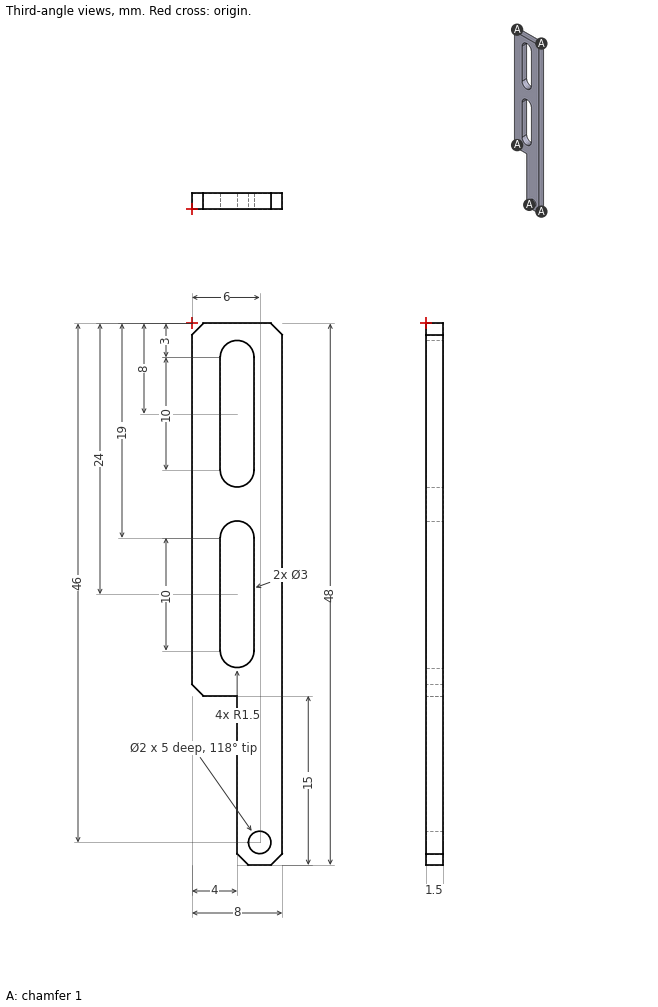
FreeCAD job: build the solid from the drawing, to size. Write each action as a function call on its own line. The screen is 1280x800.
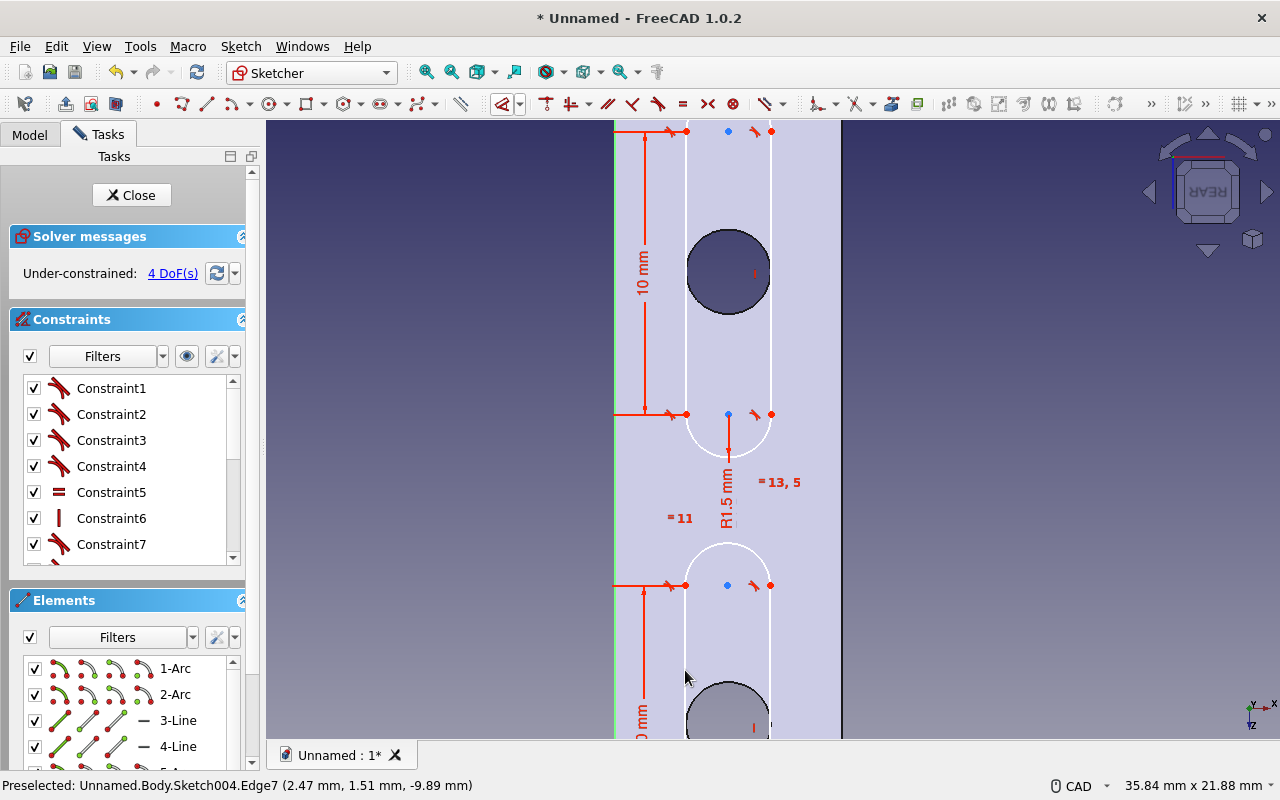
scroll(714, 356, down, 4)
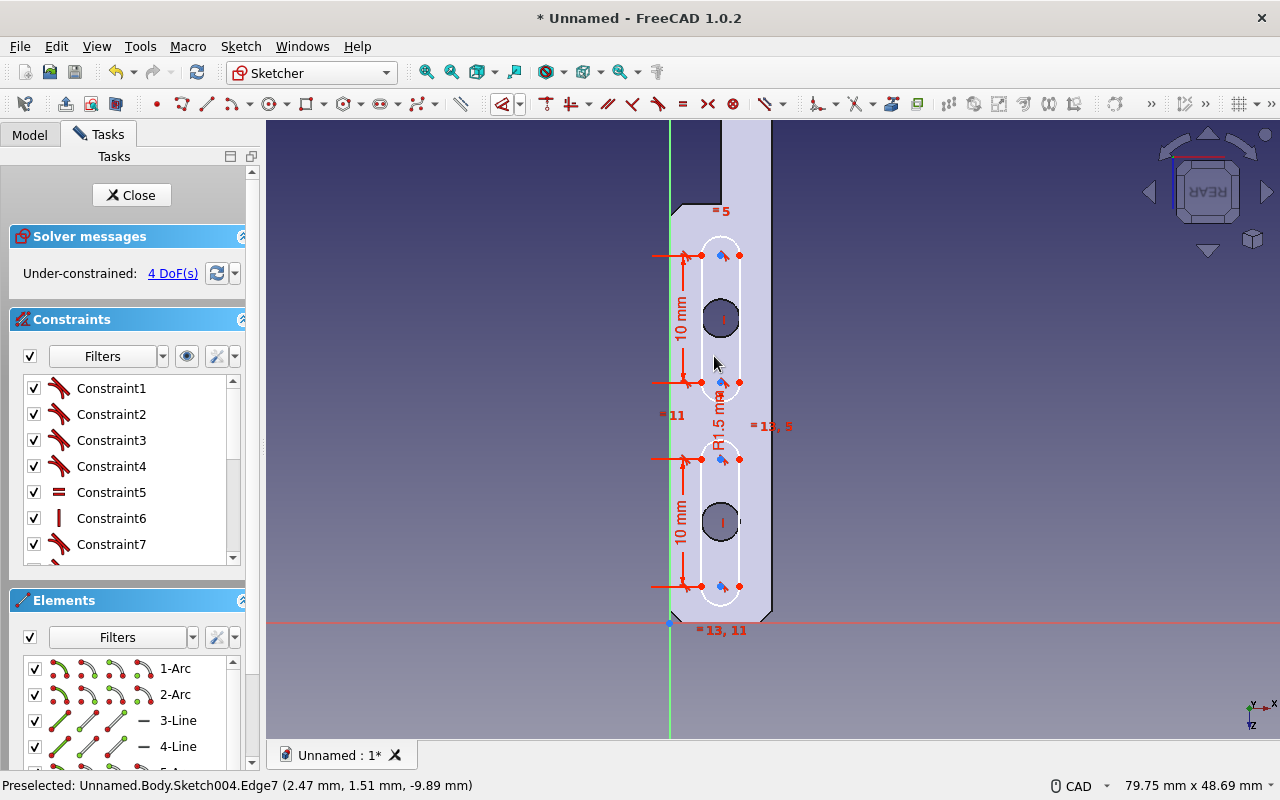
click(701, 587)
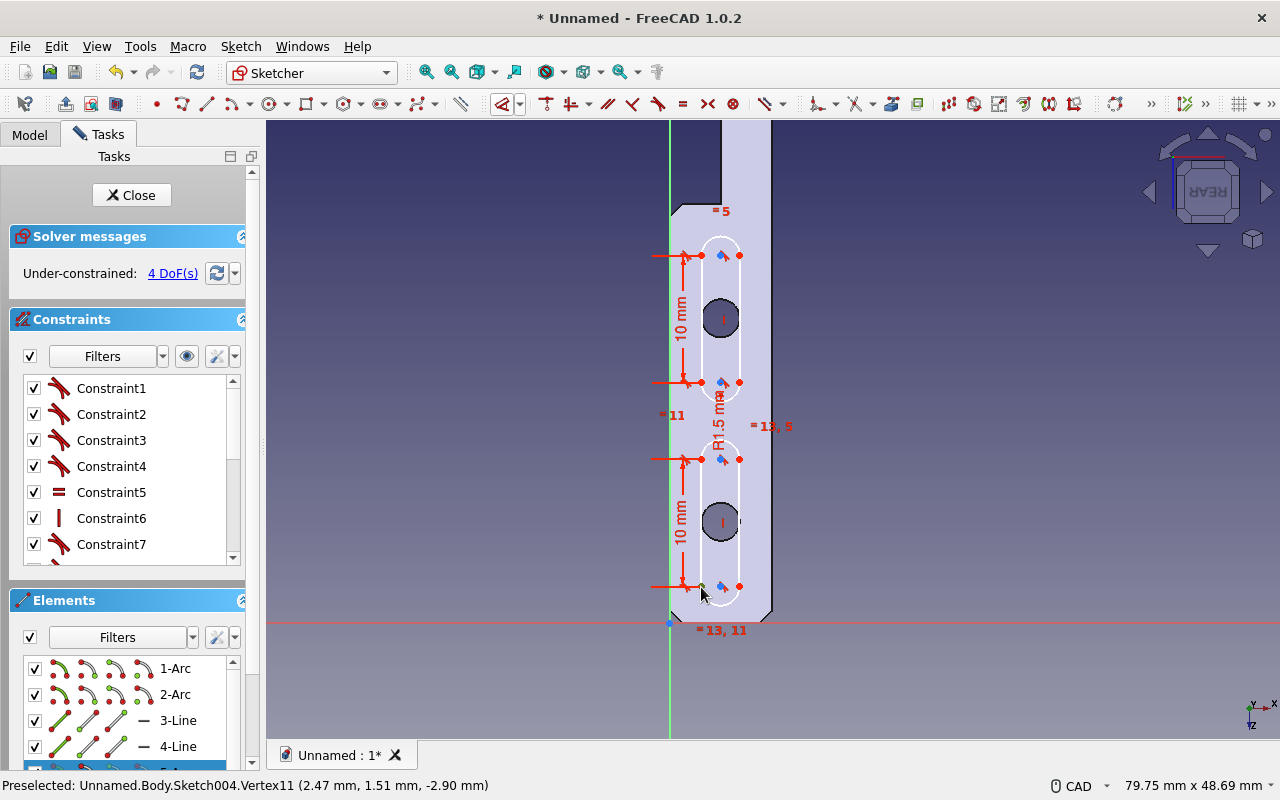
click(520, 104)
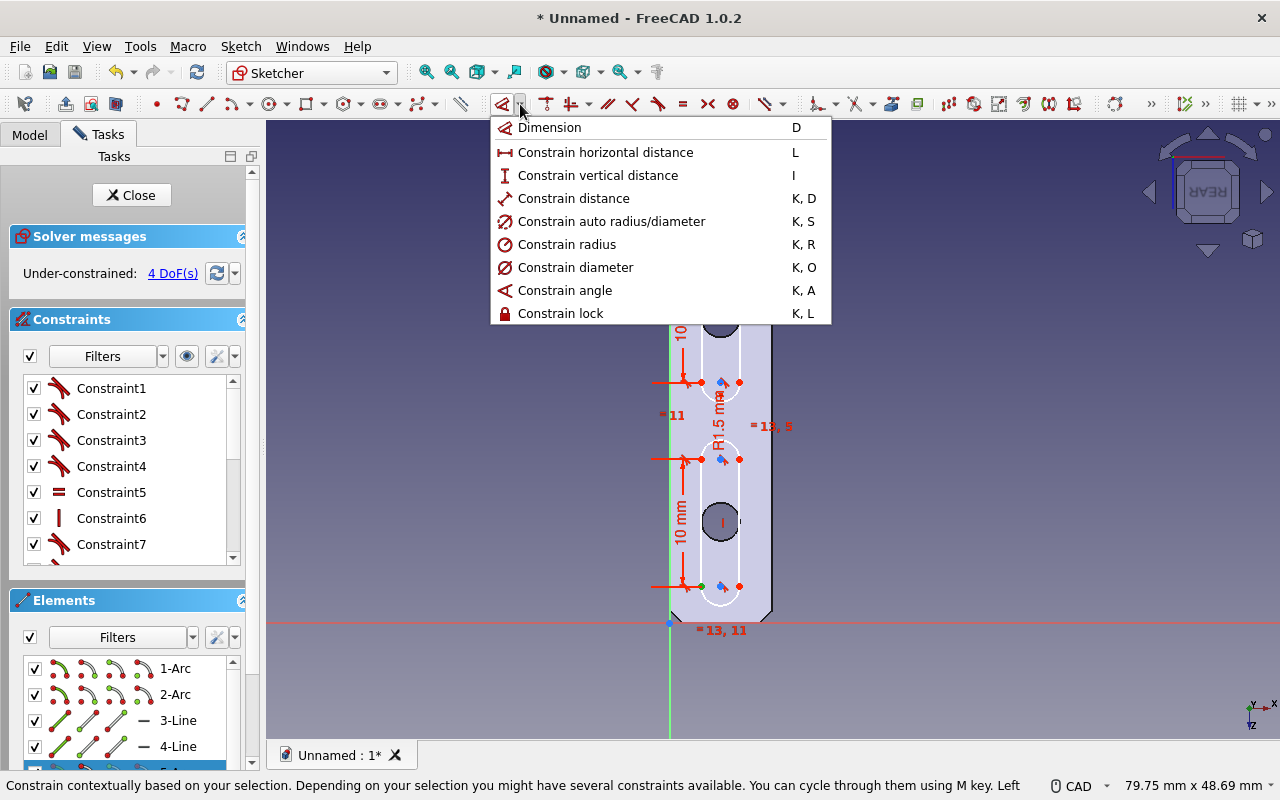
click(661, 176)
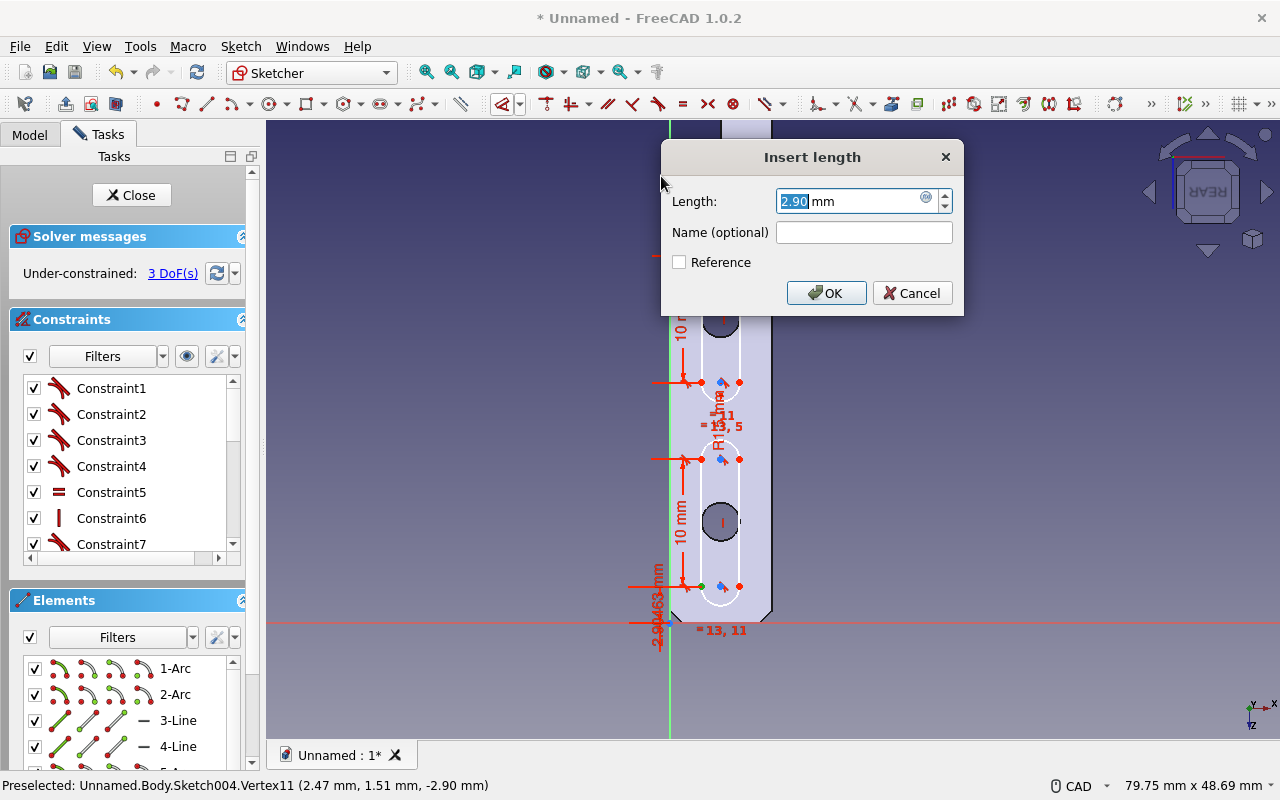
text(3)
key(Return)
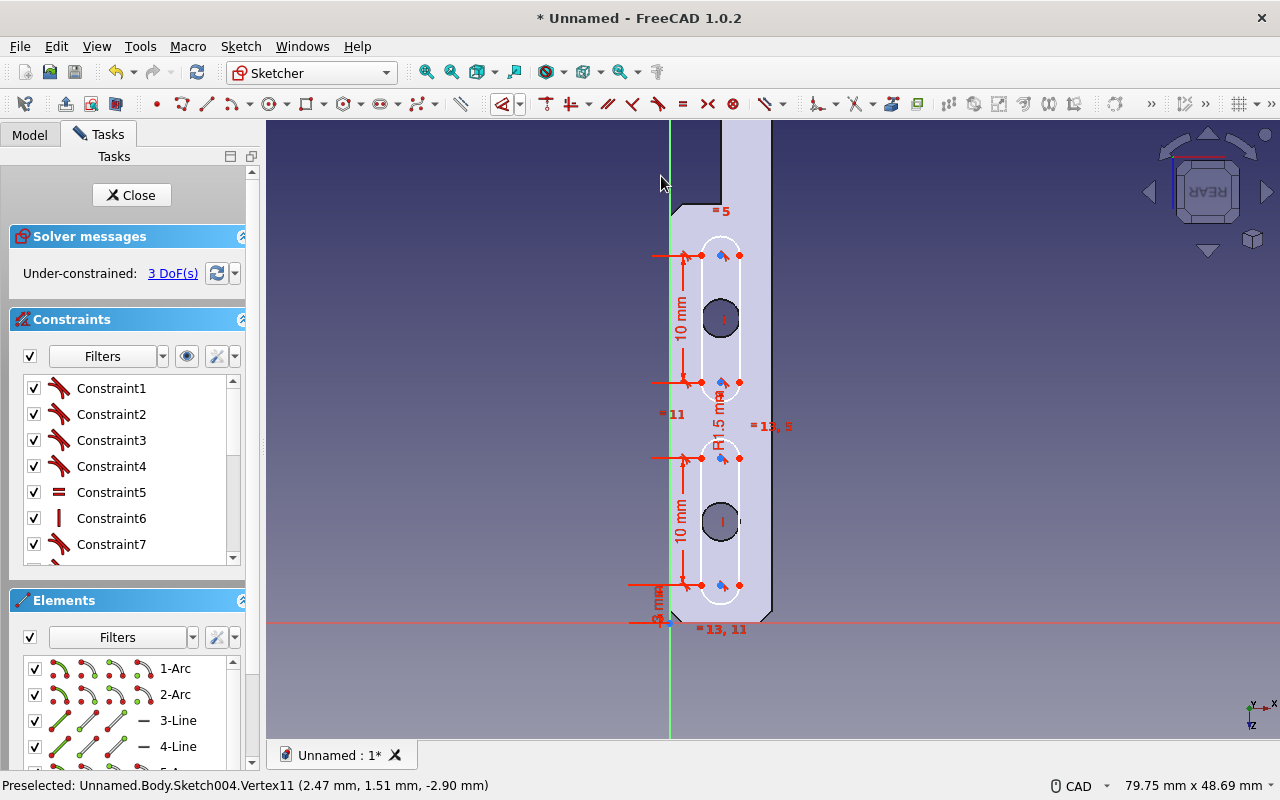
click(721, 383)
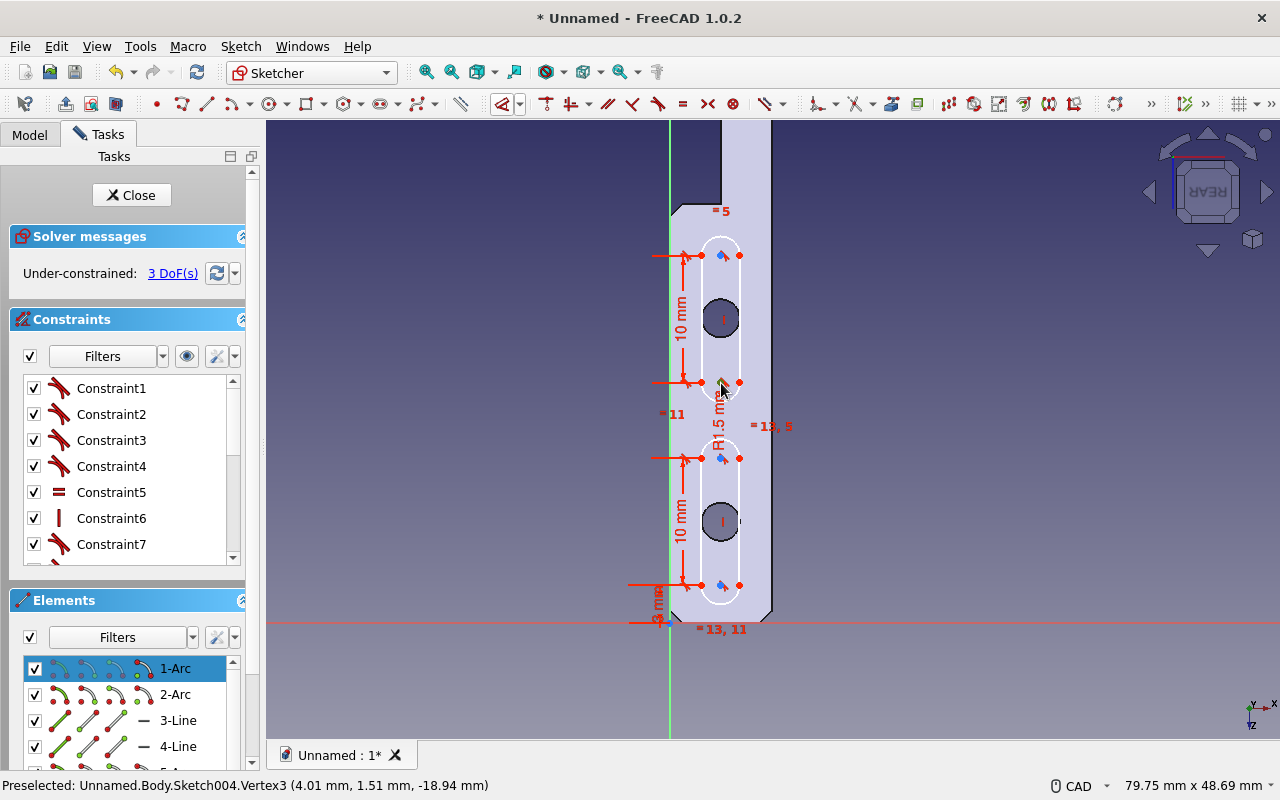
key(l)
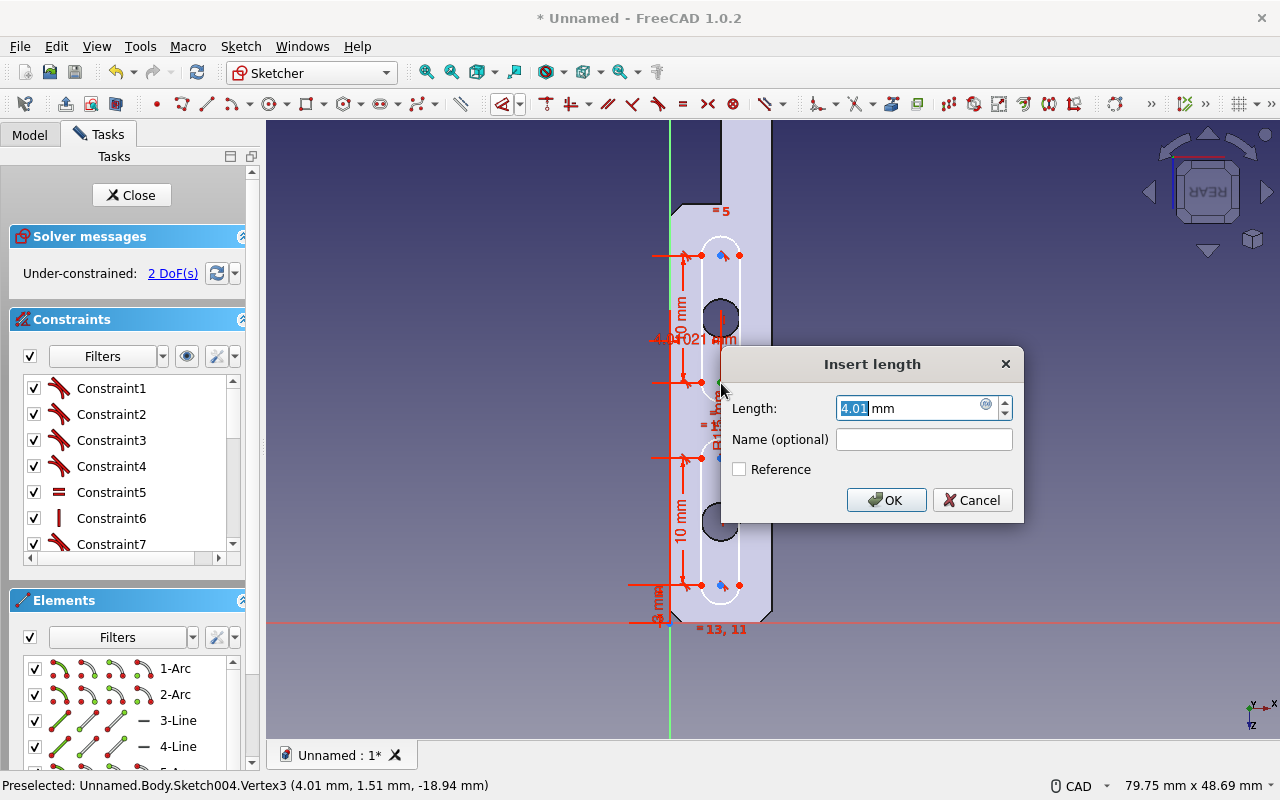
text(4)
key(Return)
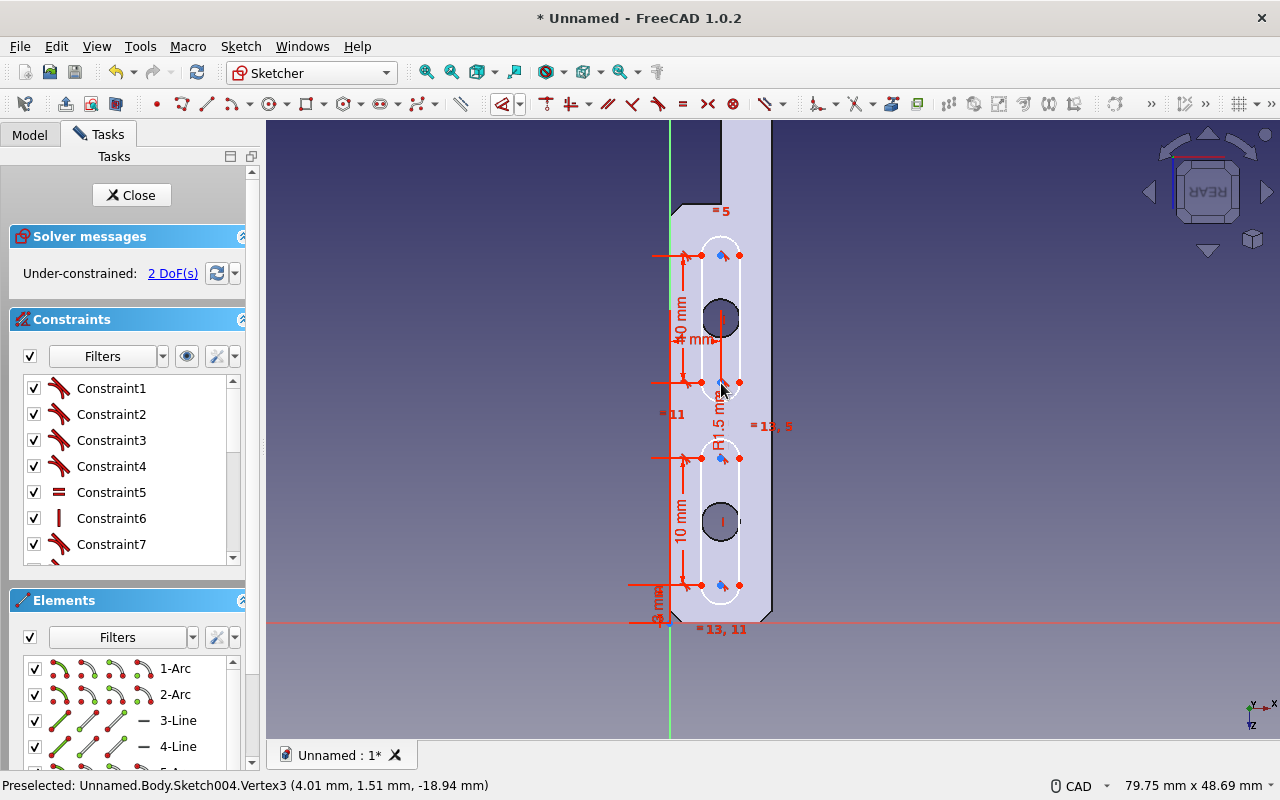
click(720, 585)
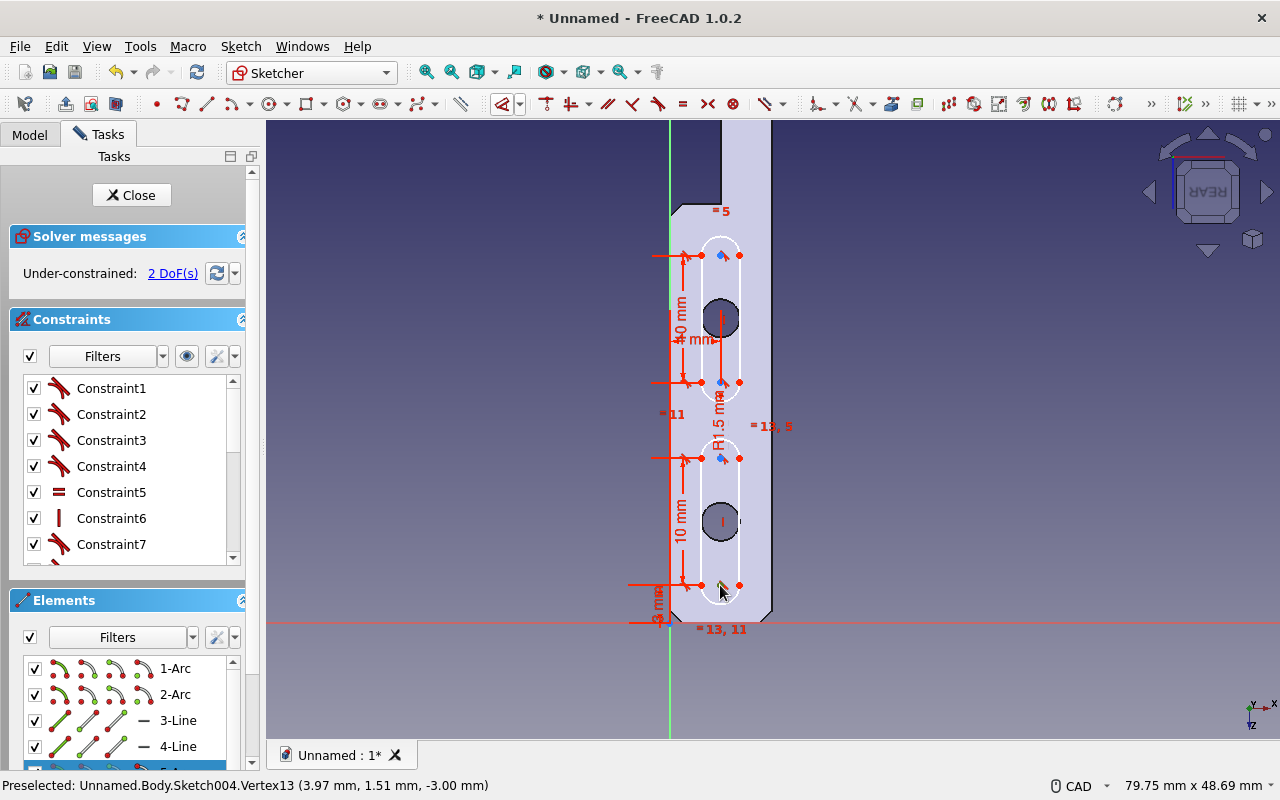
key(l)